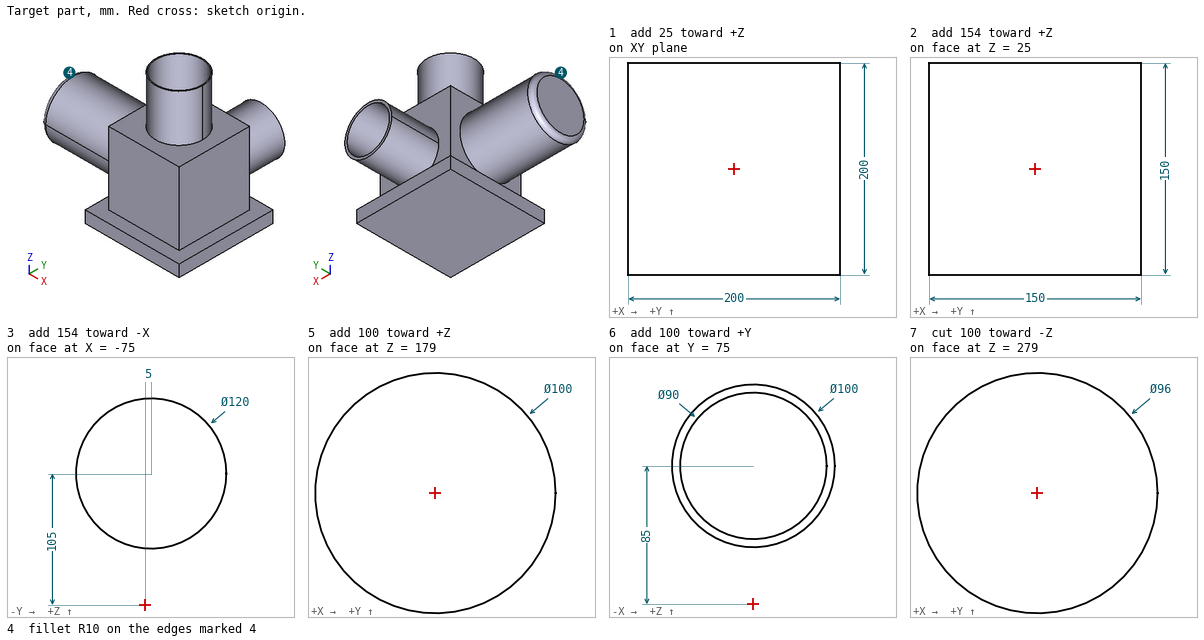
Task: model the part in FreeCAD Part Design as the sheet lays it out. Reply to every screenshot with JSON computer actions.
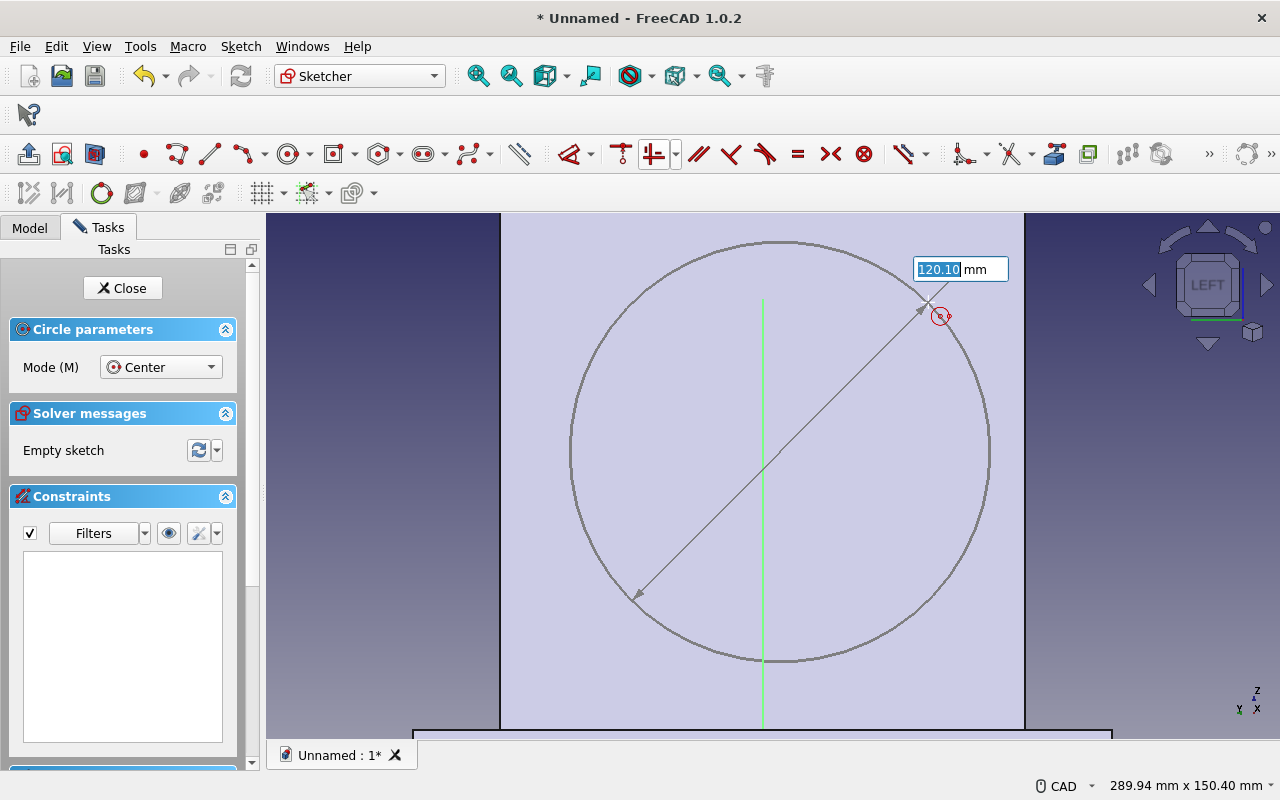
{"action": "type", "text": "120"}
{"action": "key", "text": "Return"}
{"action": "key", "text": "Escape"}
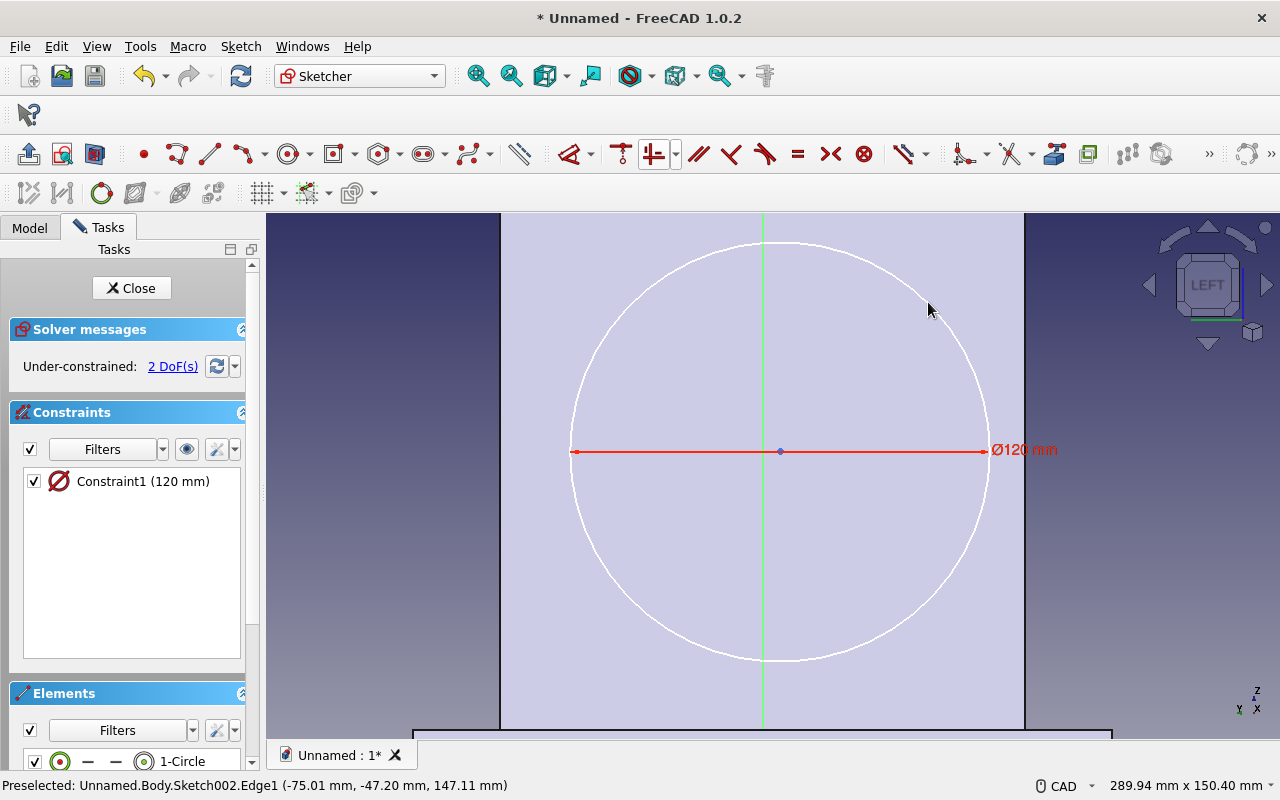
{"action": "left_click", "coordinate": [568, 154]}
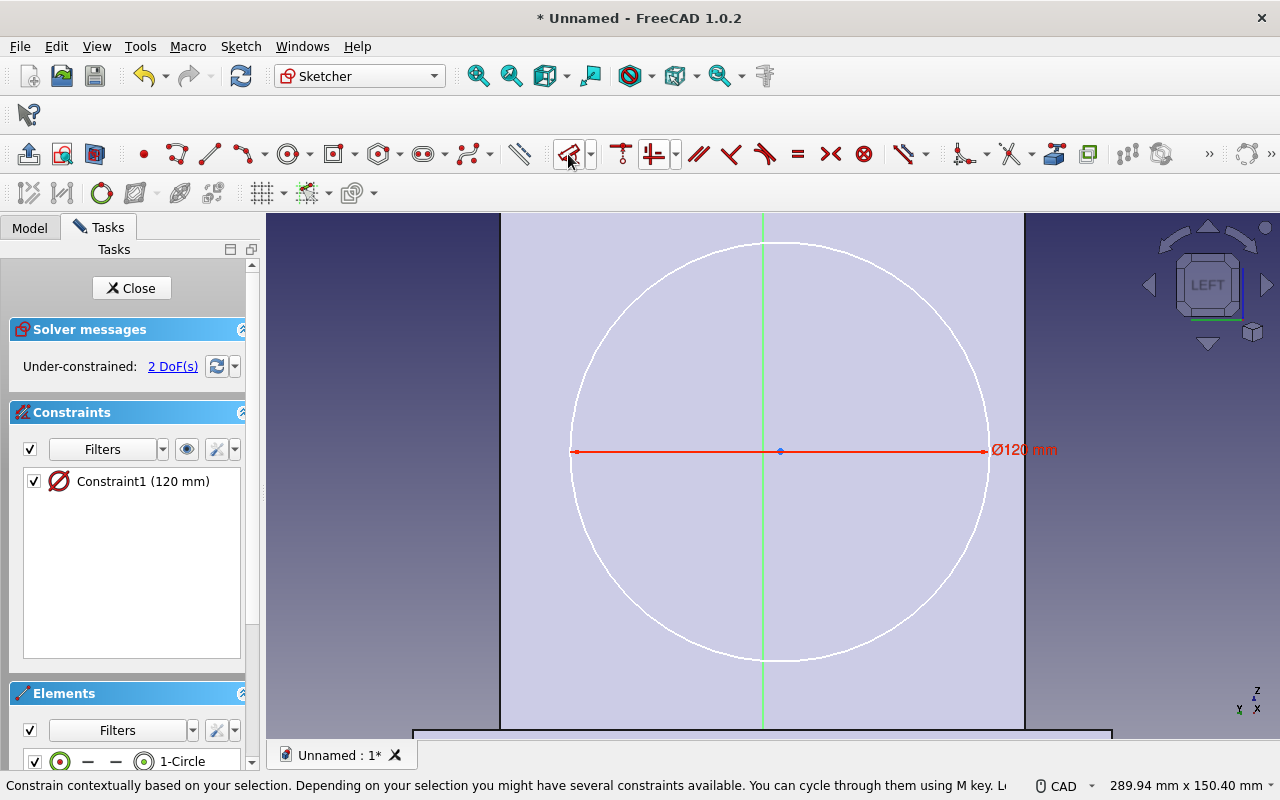
{"action": "scroll", "coordinate": [780, 452], "scroll_direction": "up", "scroll_amount": 5}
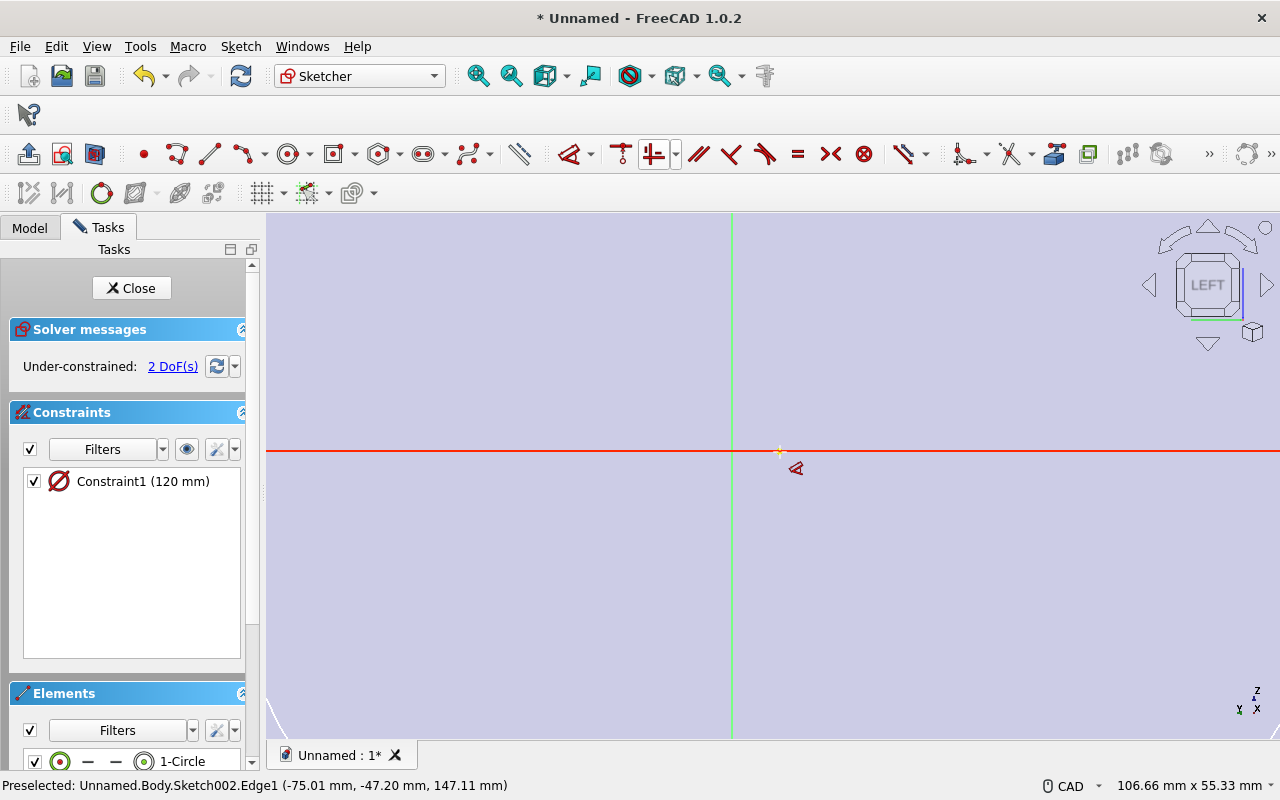
{"action": "left_click", "coordinate": [779, 451]}
{"action": "left_click", "coordinate": [755, 417]}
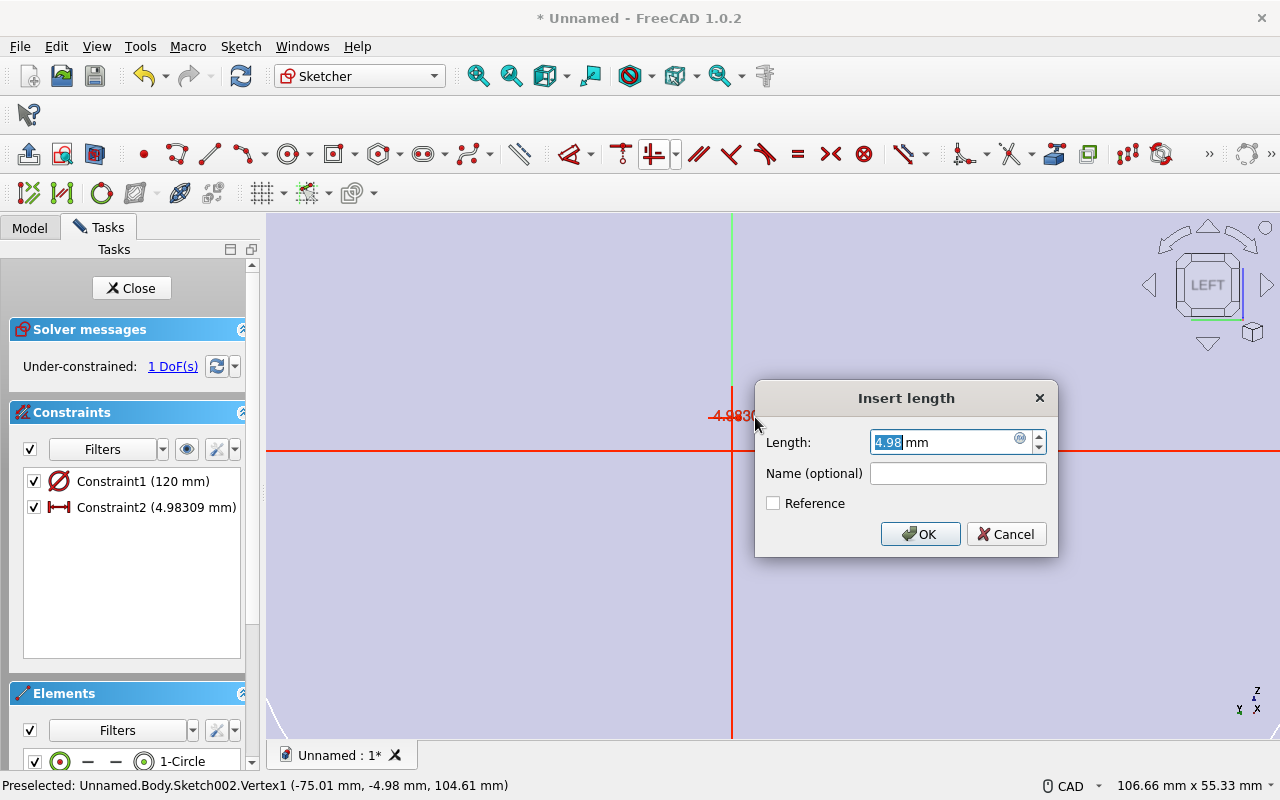
{"action": "type", "text": "5"}
{"action": "key", "text": "Return"}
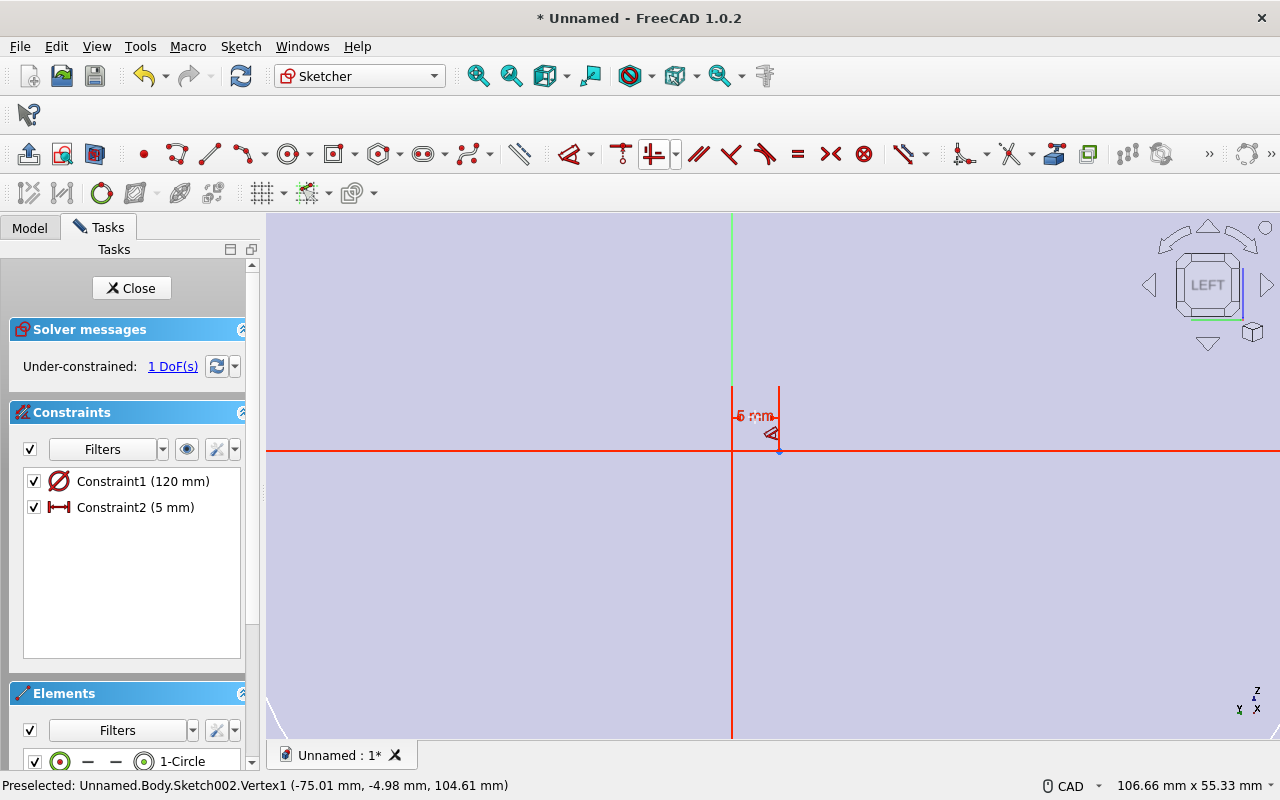
{"action": "scroll", "coordinate": [686, 429], "scroll_direction": "down", "scroll_amount": 8}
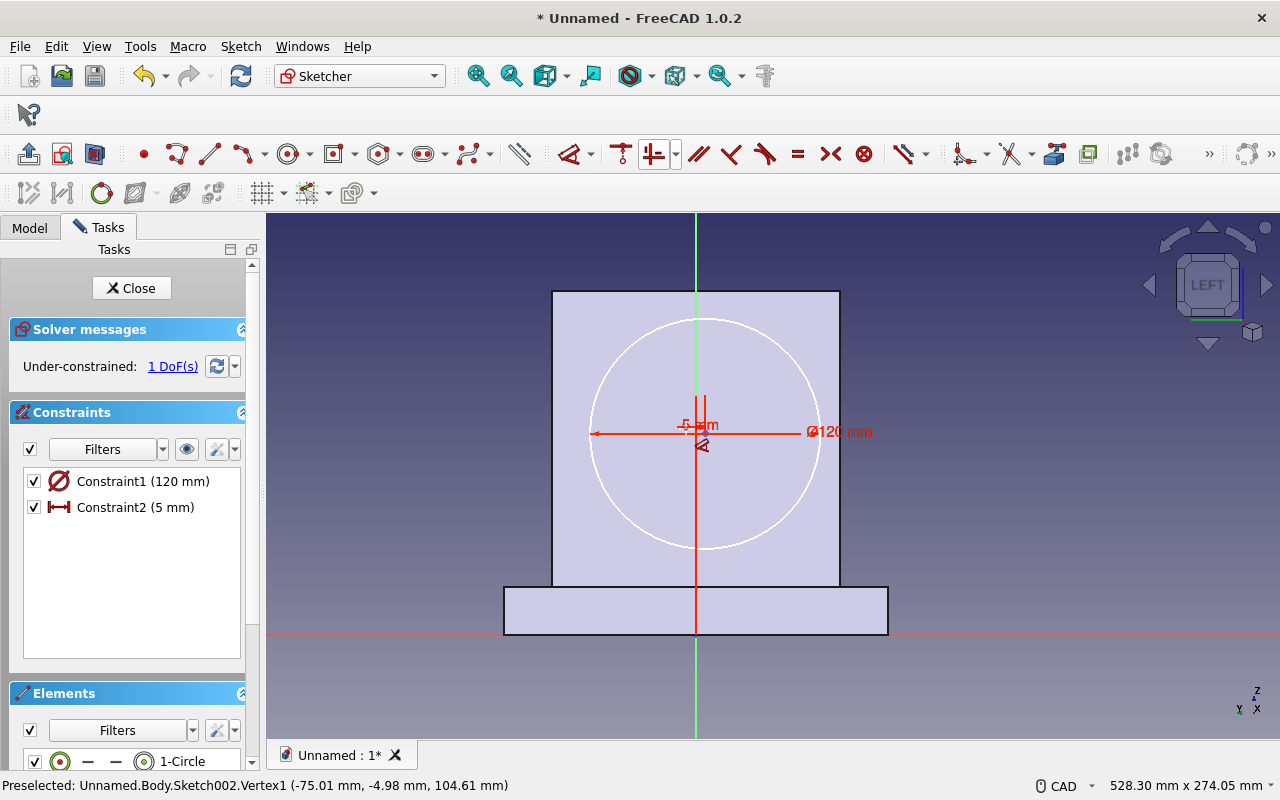
{"action": "left_click", "coordinate": [705, 434]}
{"action": "left_click", "coordinate": [662, 488]}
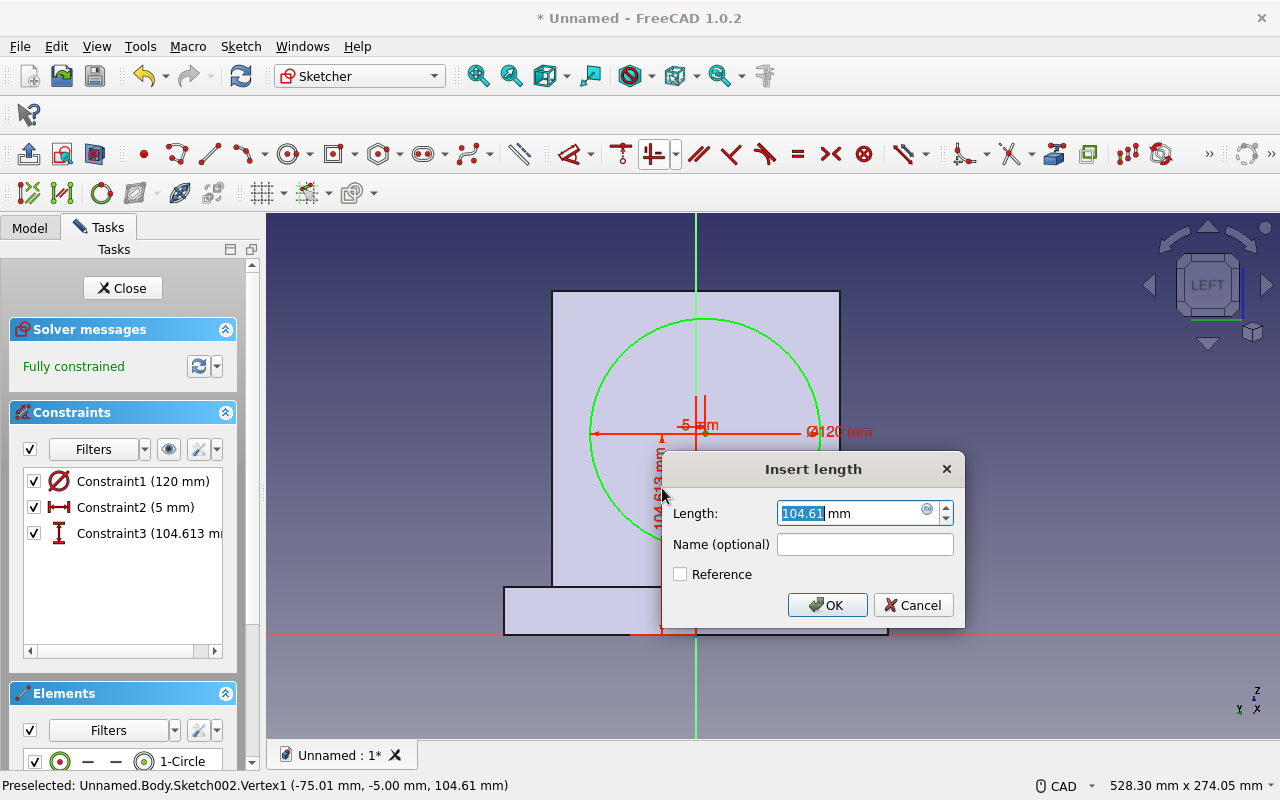
{"action": "type", "text": "105"}
{"action": "key", "text": "Return"}
{"action": "key", "text": "Escape"}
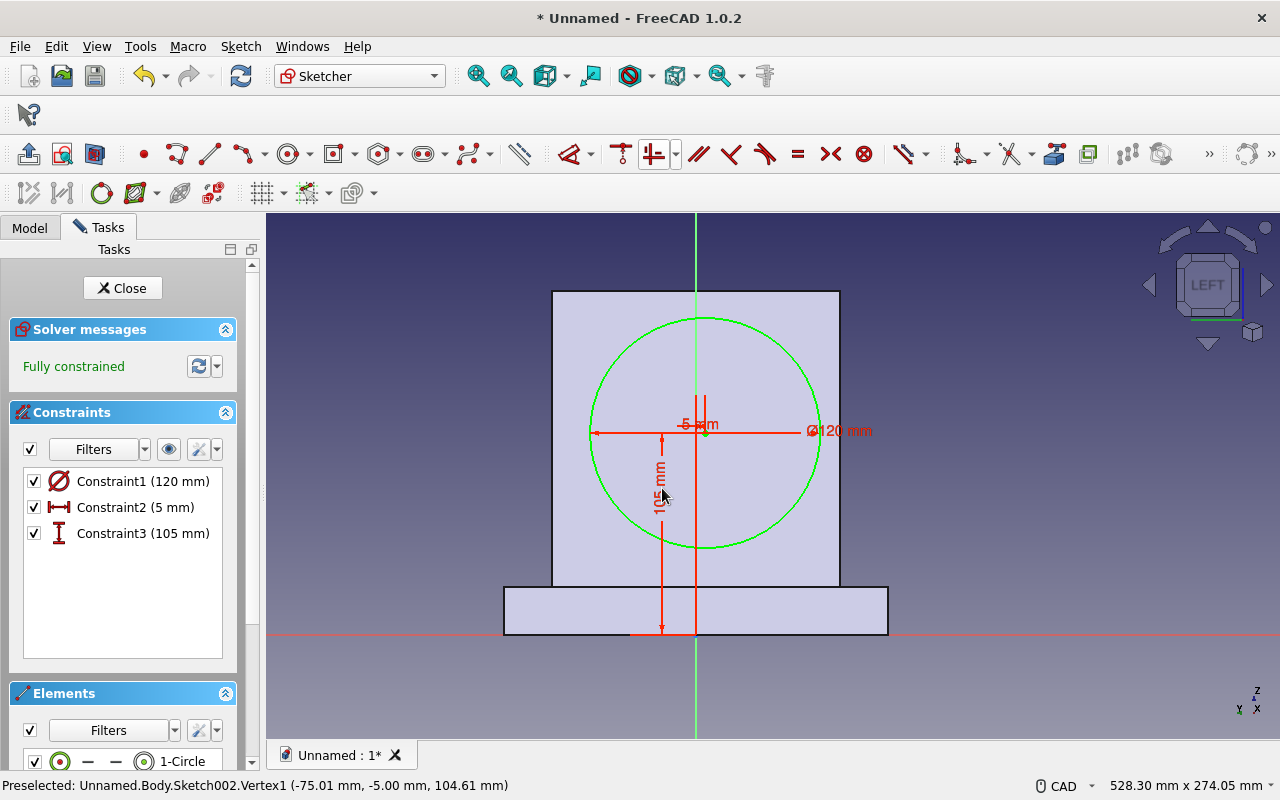
{"action": "left_click", "coordinate": [123, 288]}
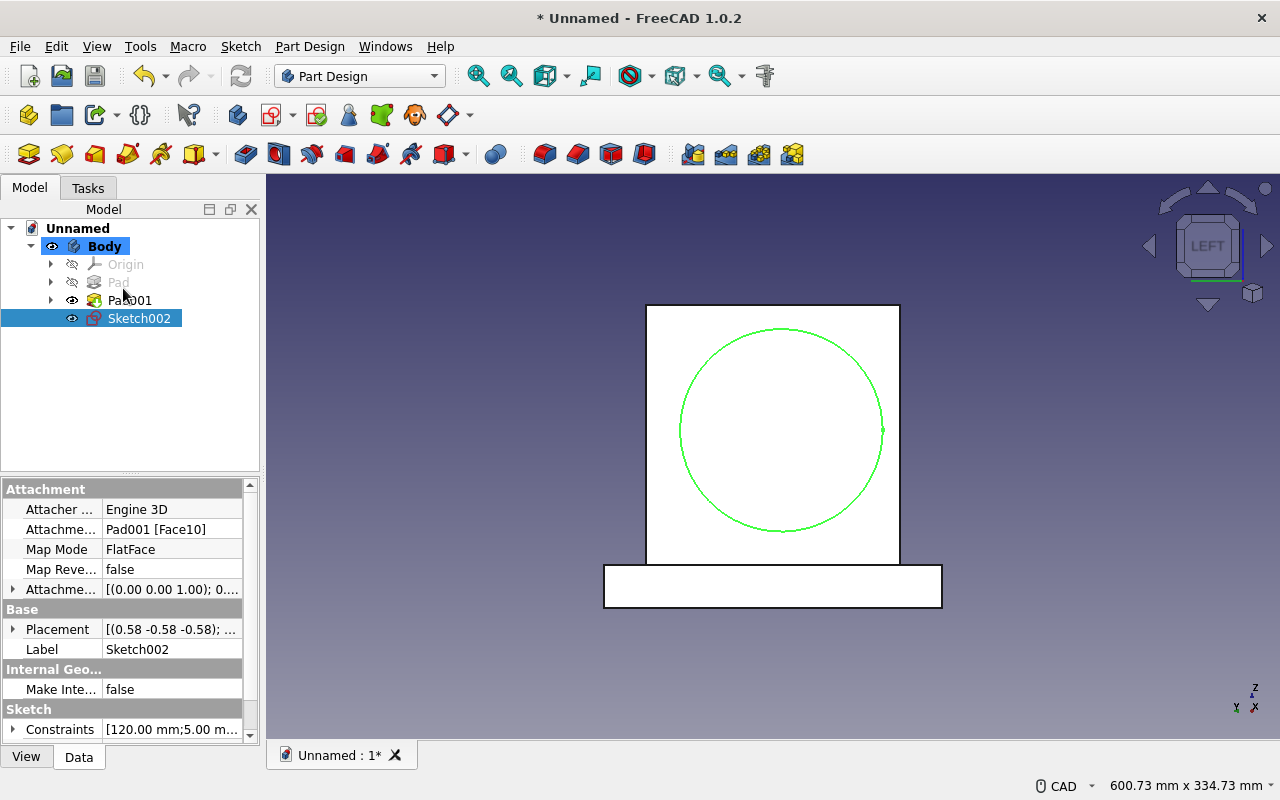
{"action": "left_click", "coordinate": [29, 154]}